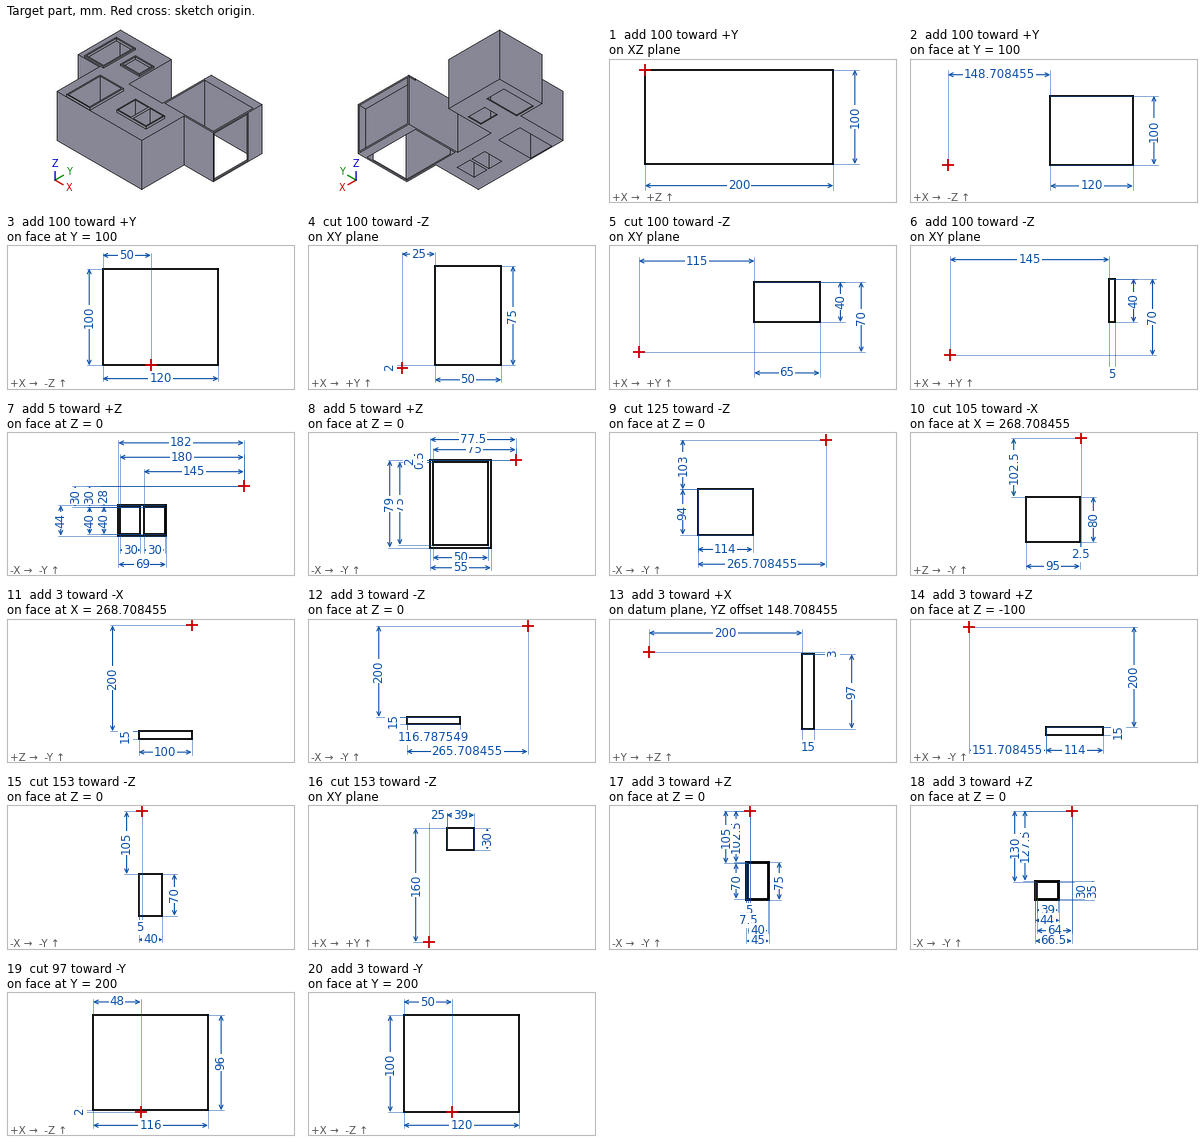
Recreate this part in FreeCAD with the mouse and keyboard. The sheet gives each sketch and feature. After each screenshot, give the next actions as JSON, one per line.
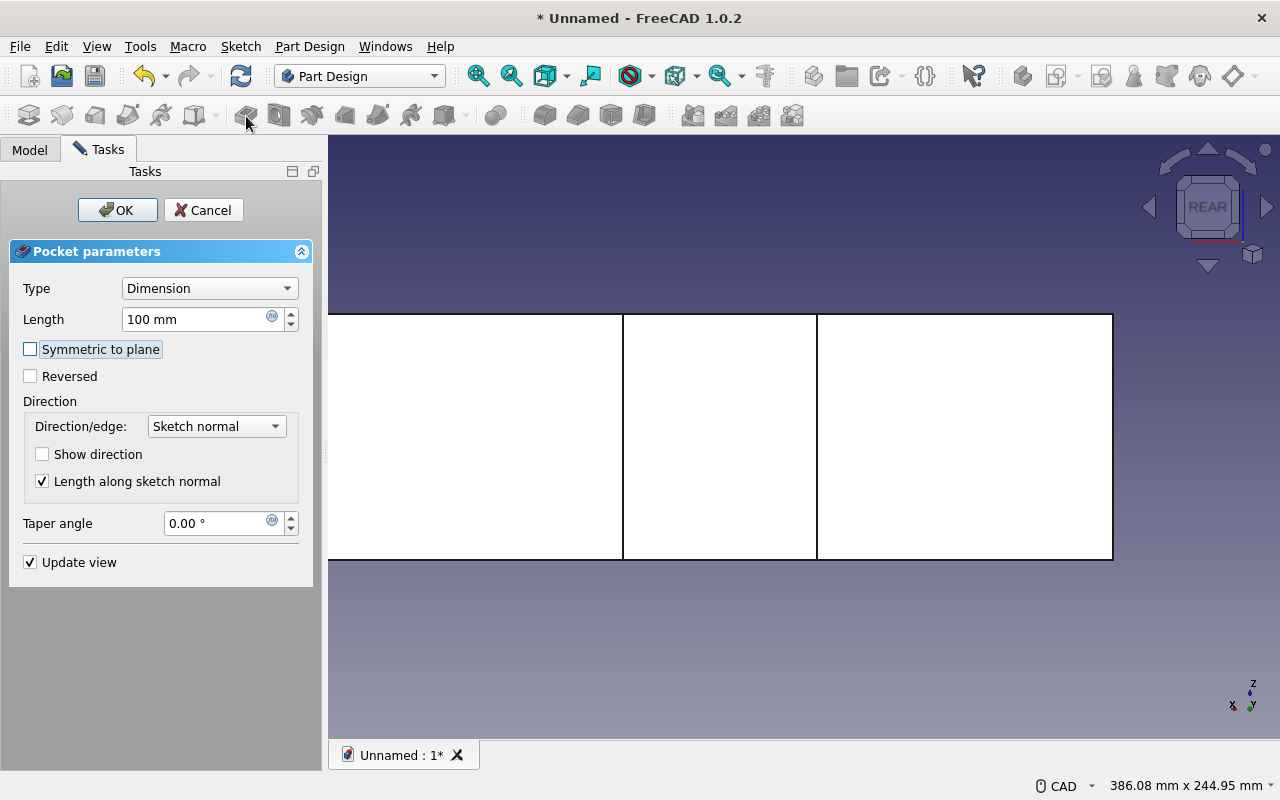
{"action": "left_click", "coordinate": [118, 210]}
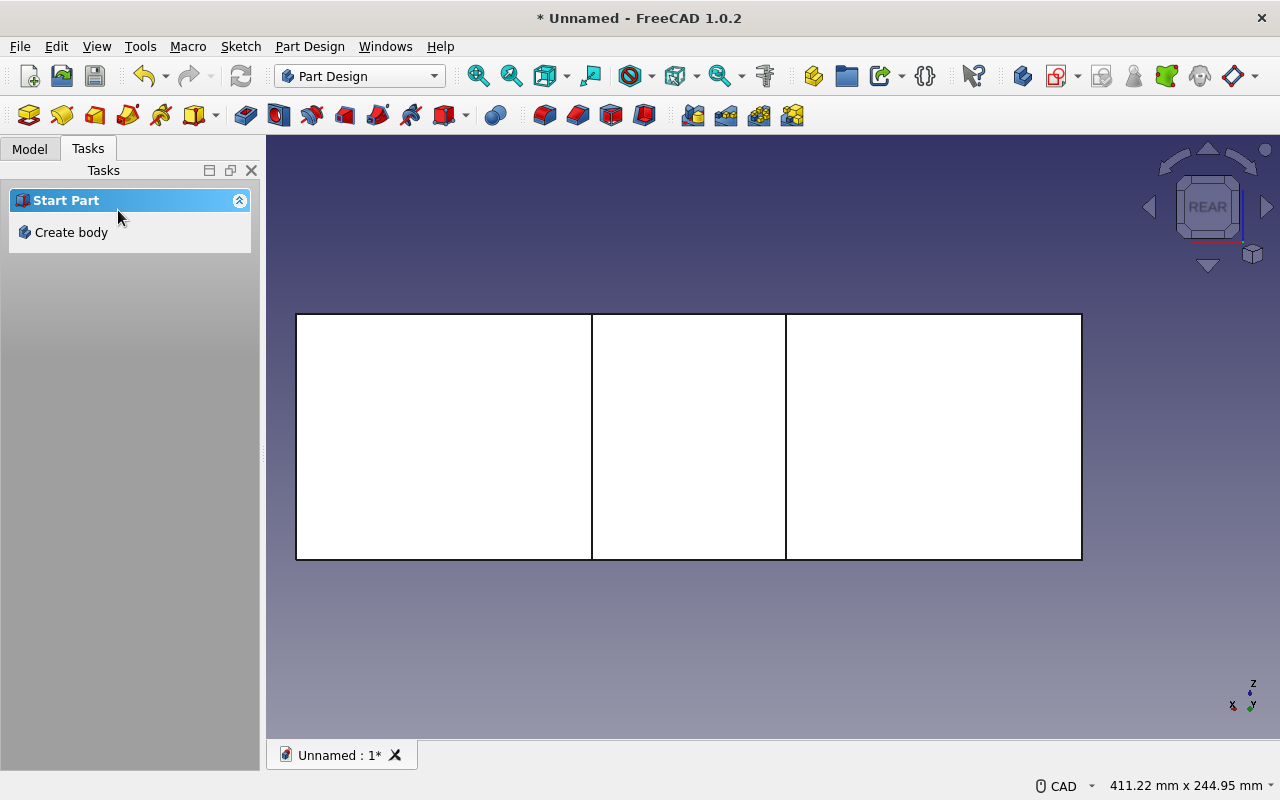
{"action": "left_click", "coordinate": [1056, 76]}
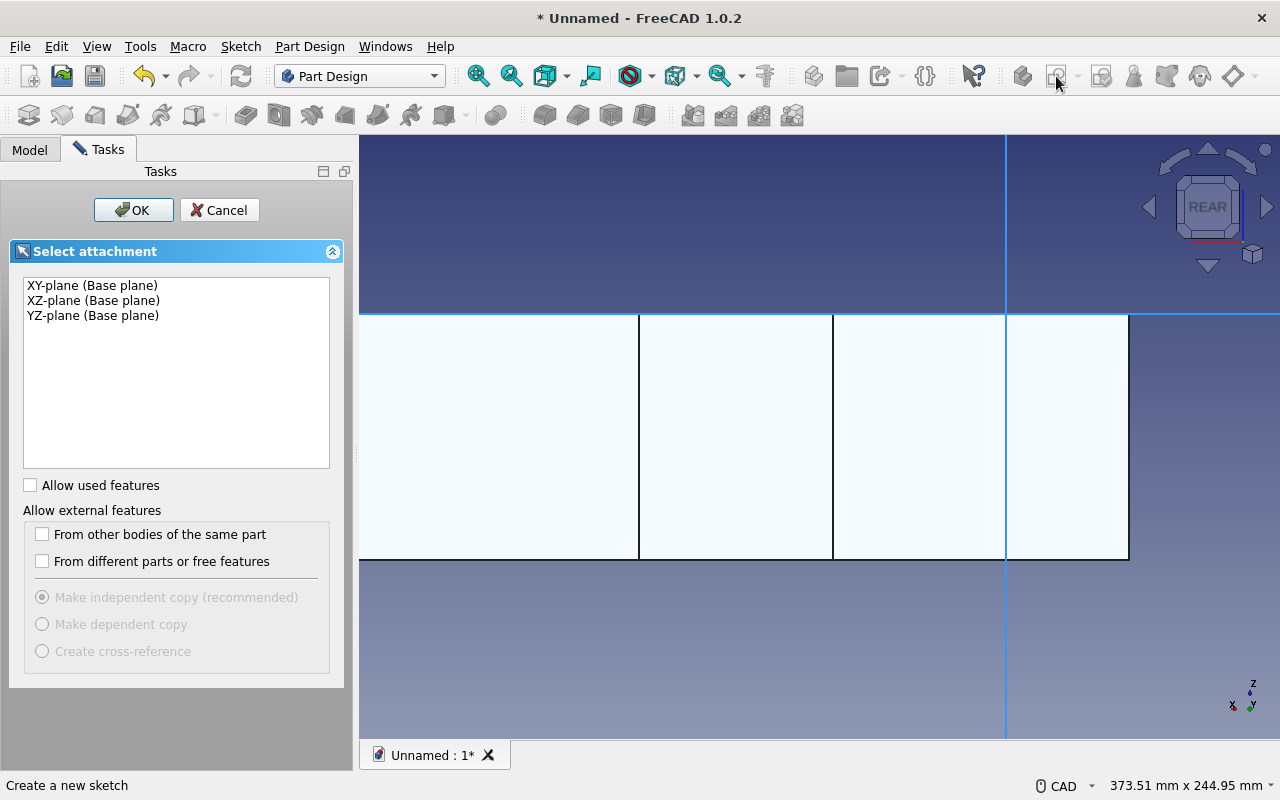
{"action": "left_click", "coordinate": [84, 286]}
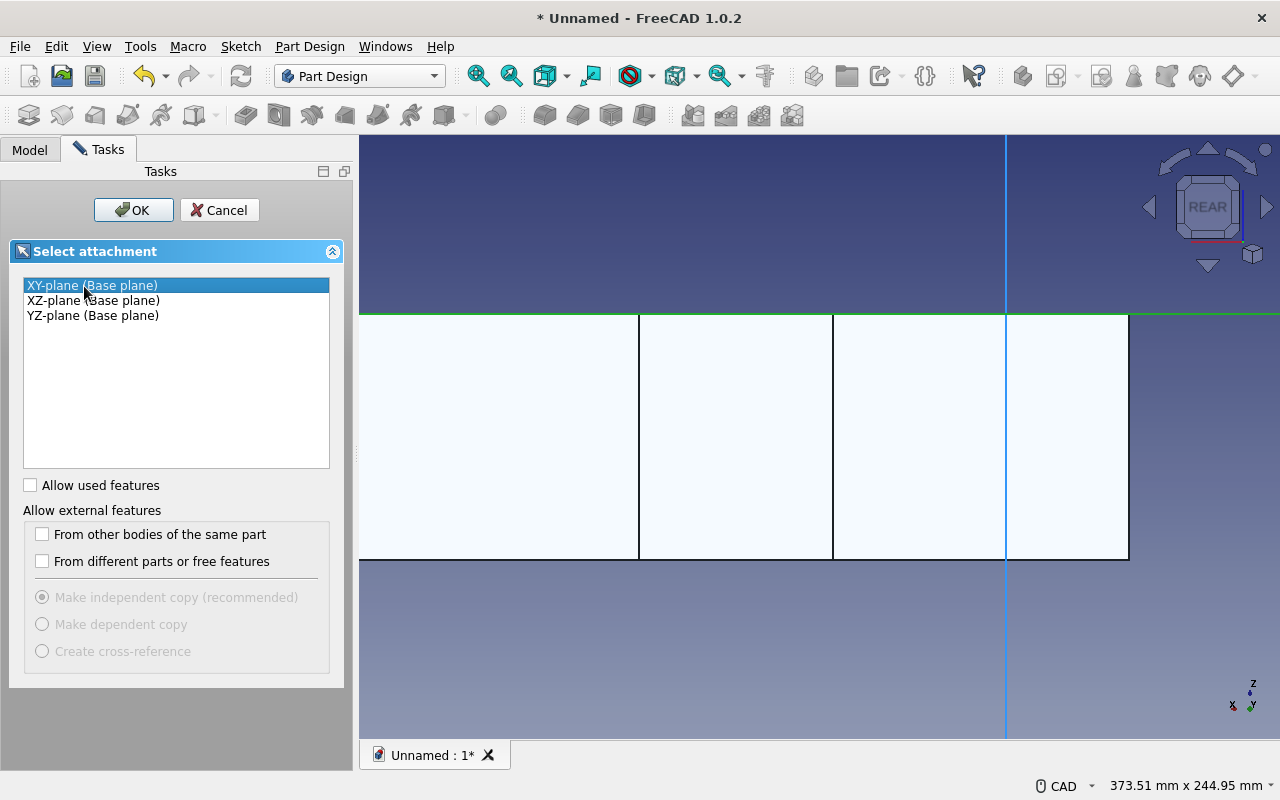
{"action": "left_click", "coordinate": [134, 210]}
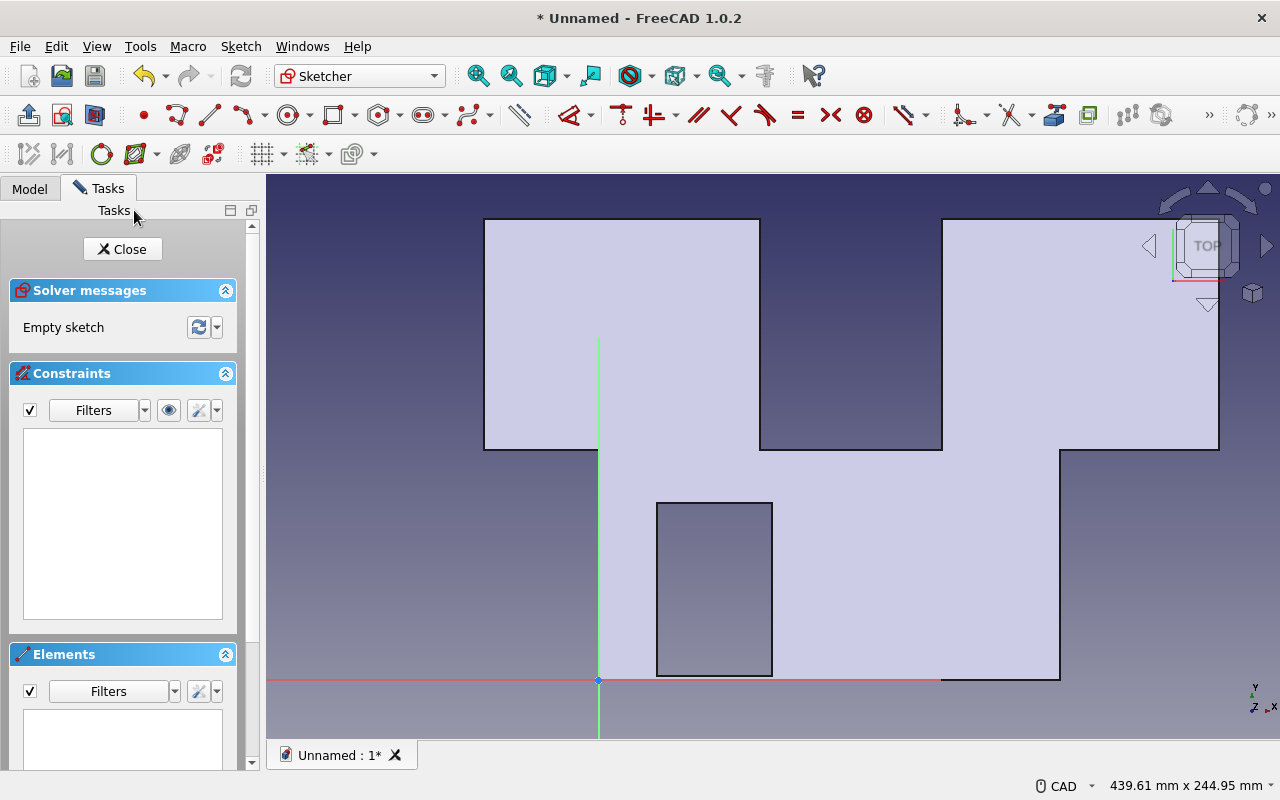
{"action": "scroll", "coordinate": [1016, 600], "scroll_direction": "up", "scroll_amount": 7}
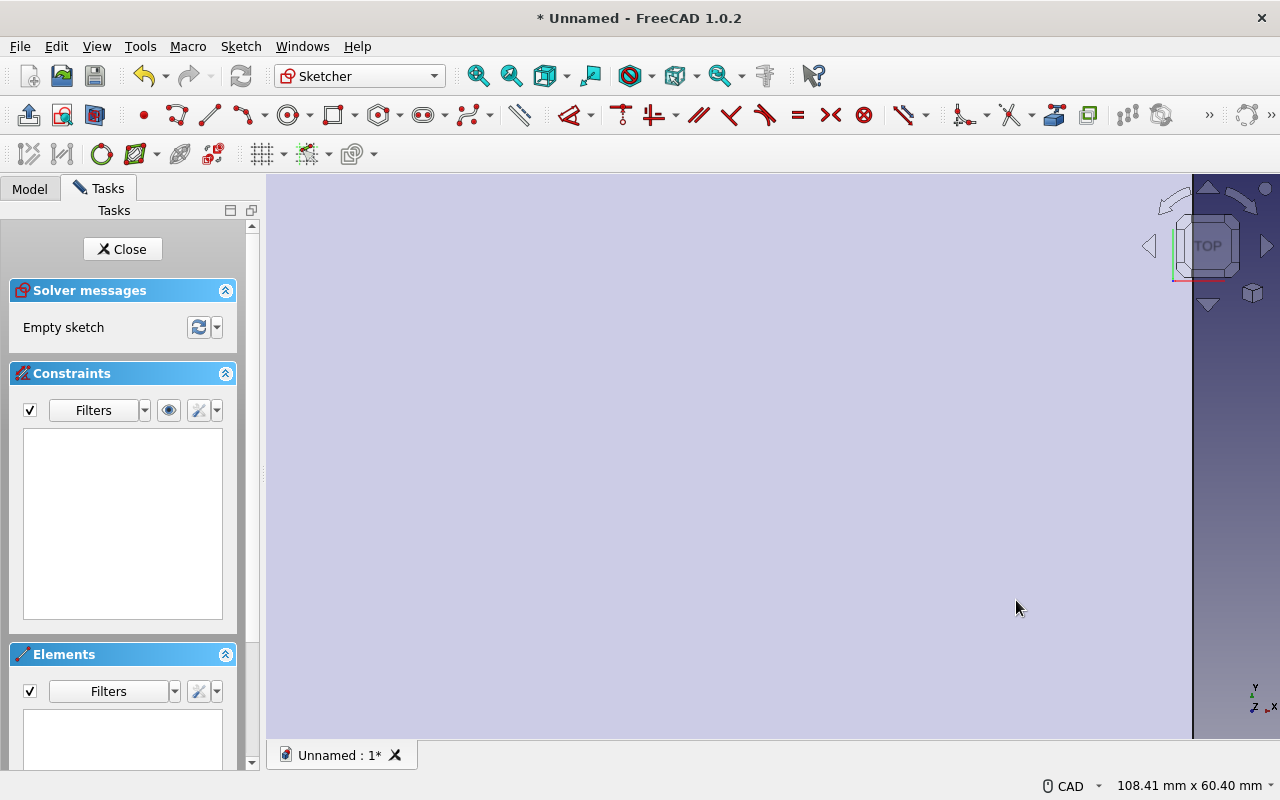
{"action": "left_click", "coordinate": [332, 116]}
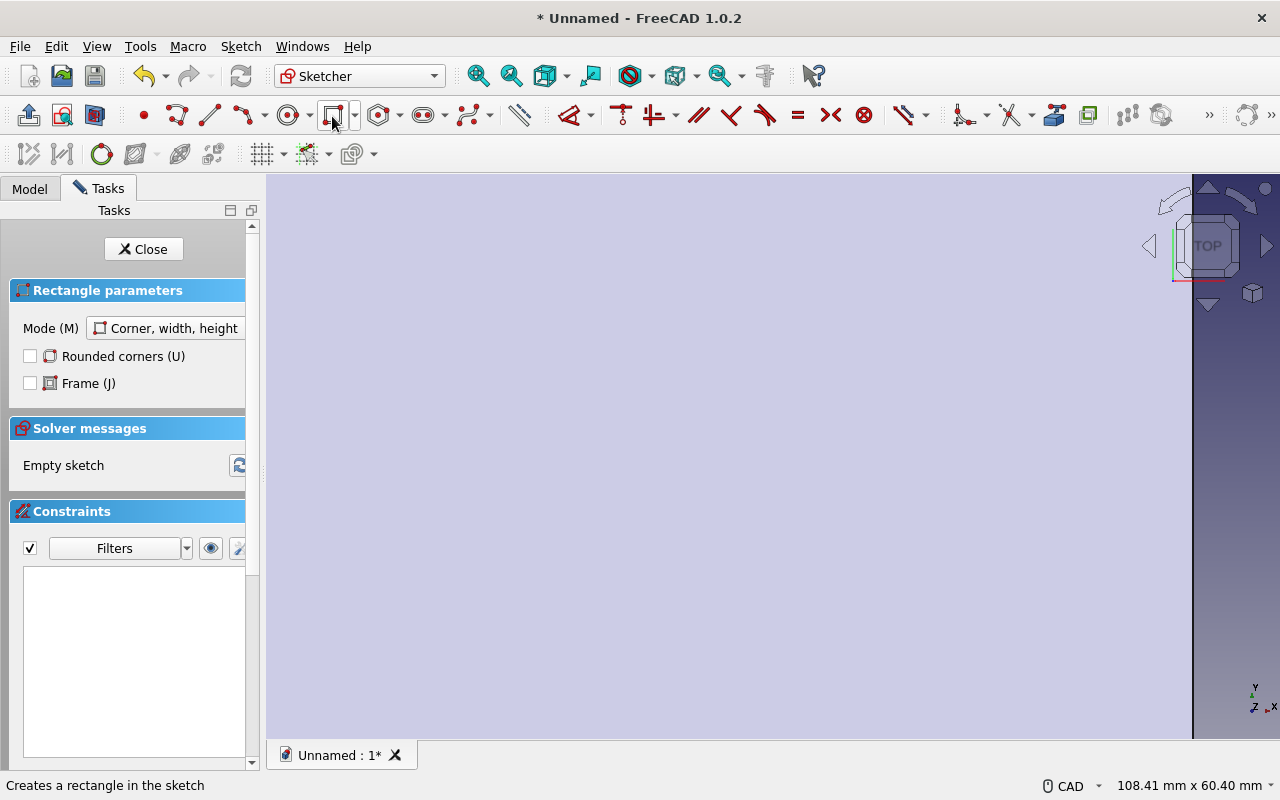
{"action": "left_click", "coordinate": [398, 269]}
{"action": "mouse_move", "coordinate": [1006, 643]}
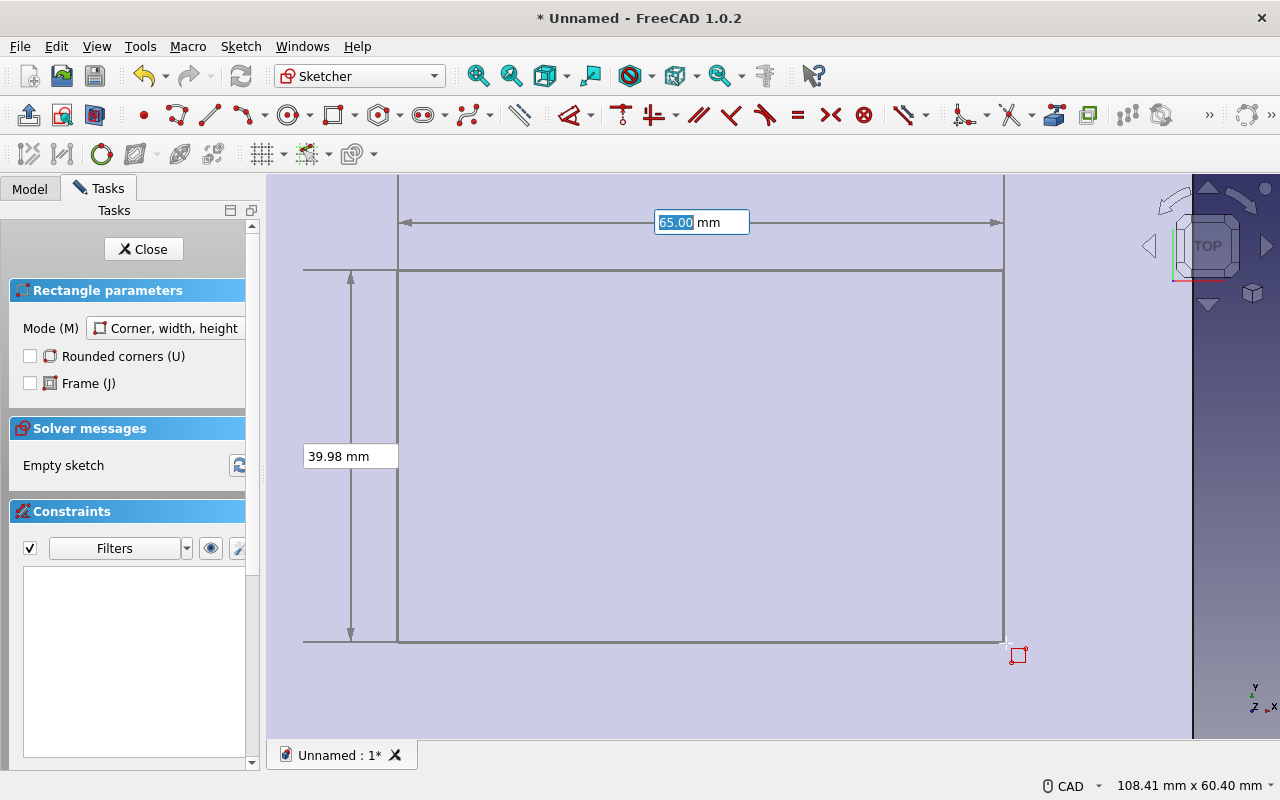
{"action": "type", "text": "65"}
{"action": "key", "text": "Tab"}
{"action": "type", "text": "40"}
{"action": "key", "text": "Return"}
{"action": "key", "text": "Escape"}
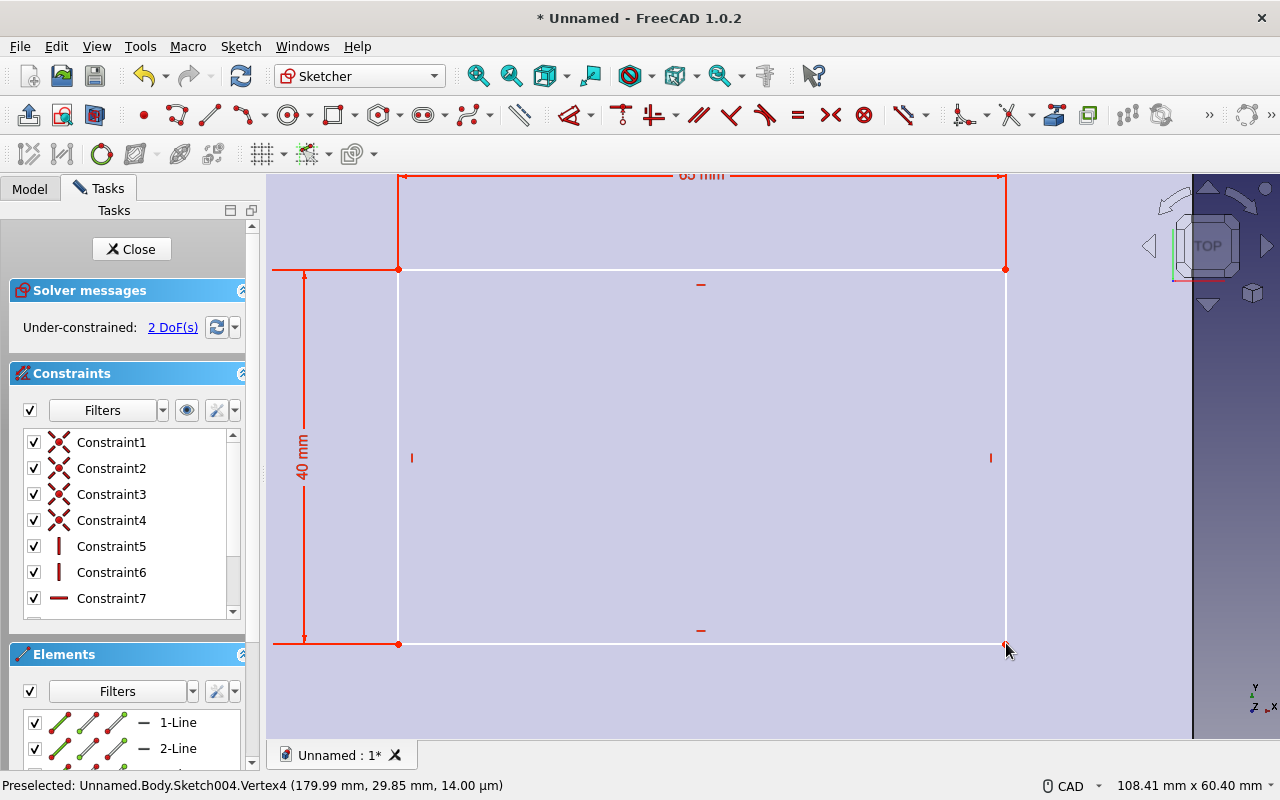
{"action": "left_click", "coordinate": [568, 116]}